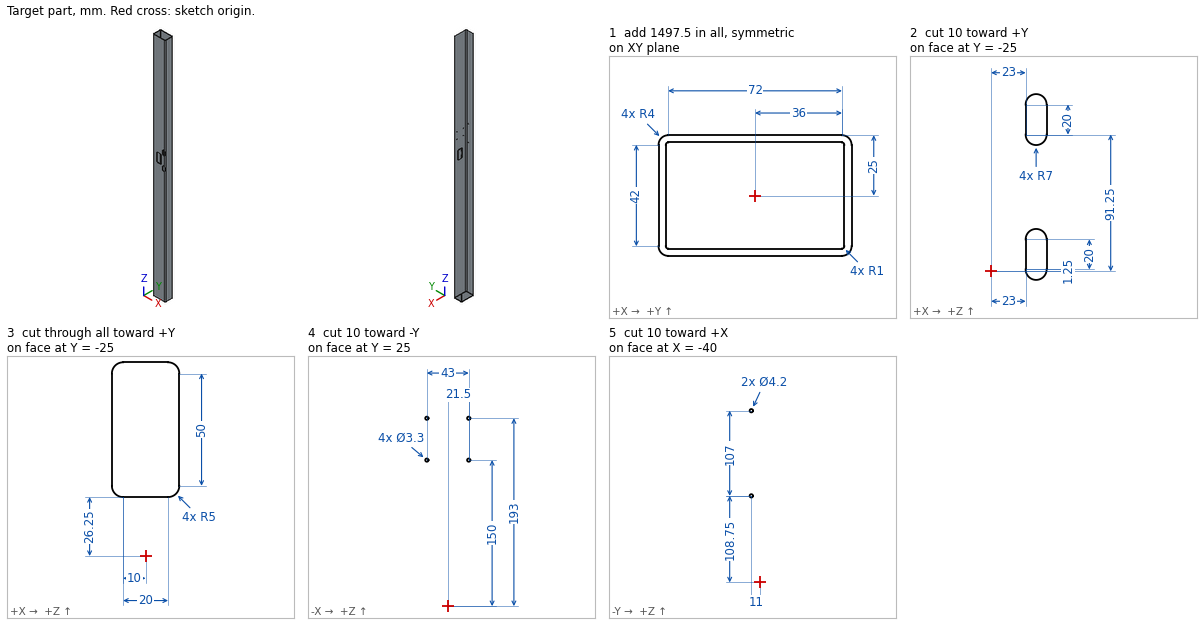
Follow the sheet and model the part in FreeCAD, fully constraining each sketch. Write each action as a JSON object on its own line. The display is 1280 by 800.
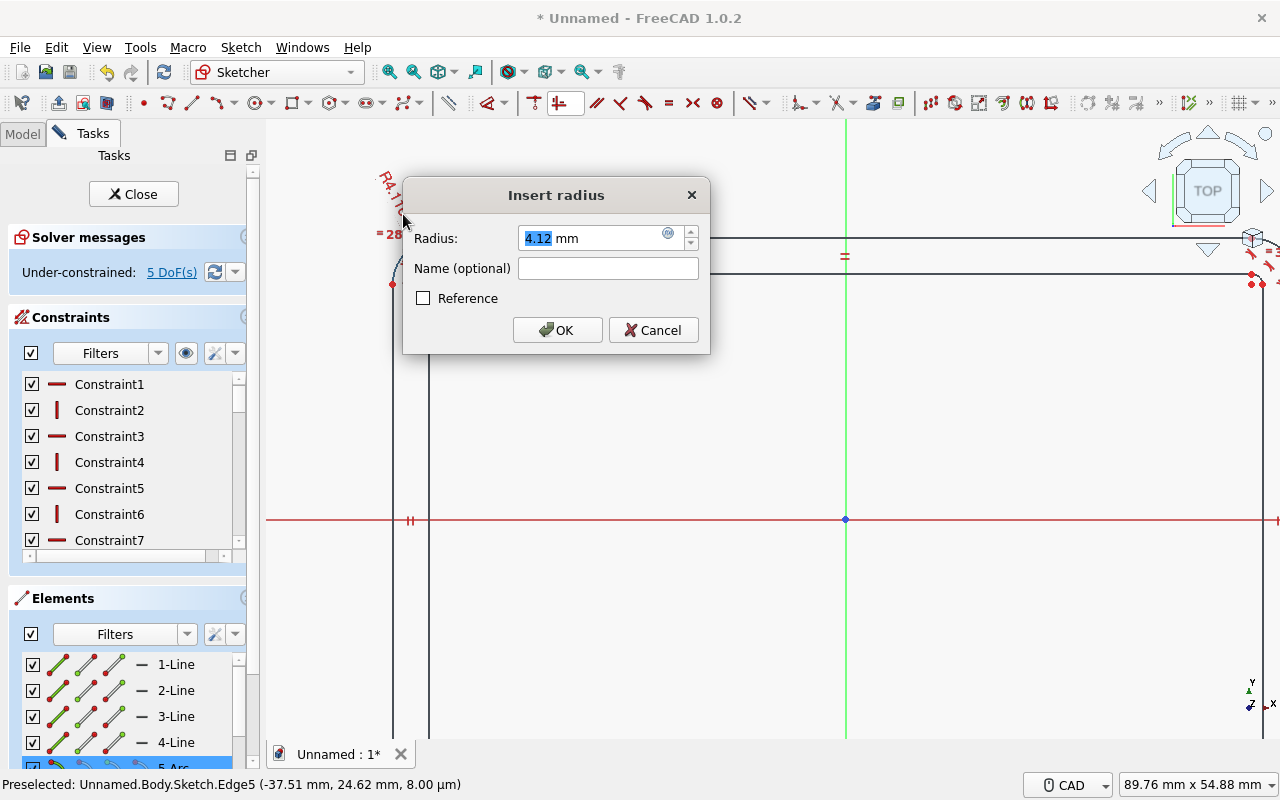
{"action": "type", "text": "4"}
{"action": "key", "text": "Return"}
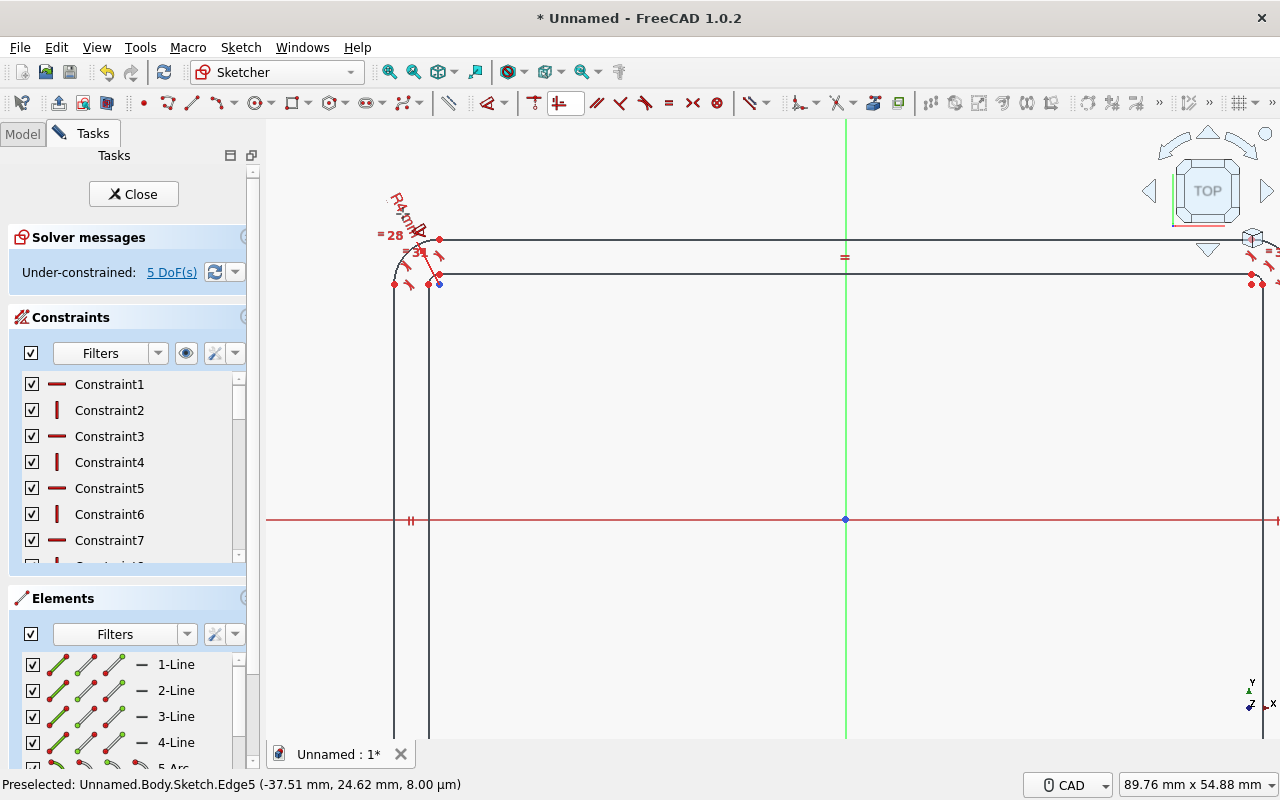
{"action": "scroll", "coordinate": [417, 245], "scroll_direction": "down", "scroll_amount": 2}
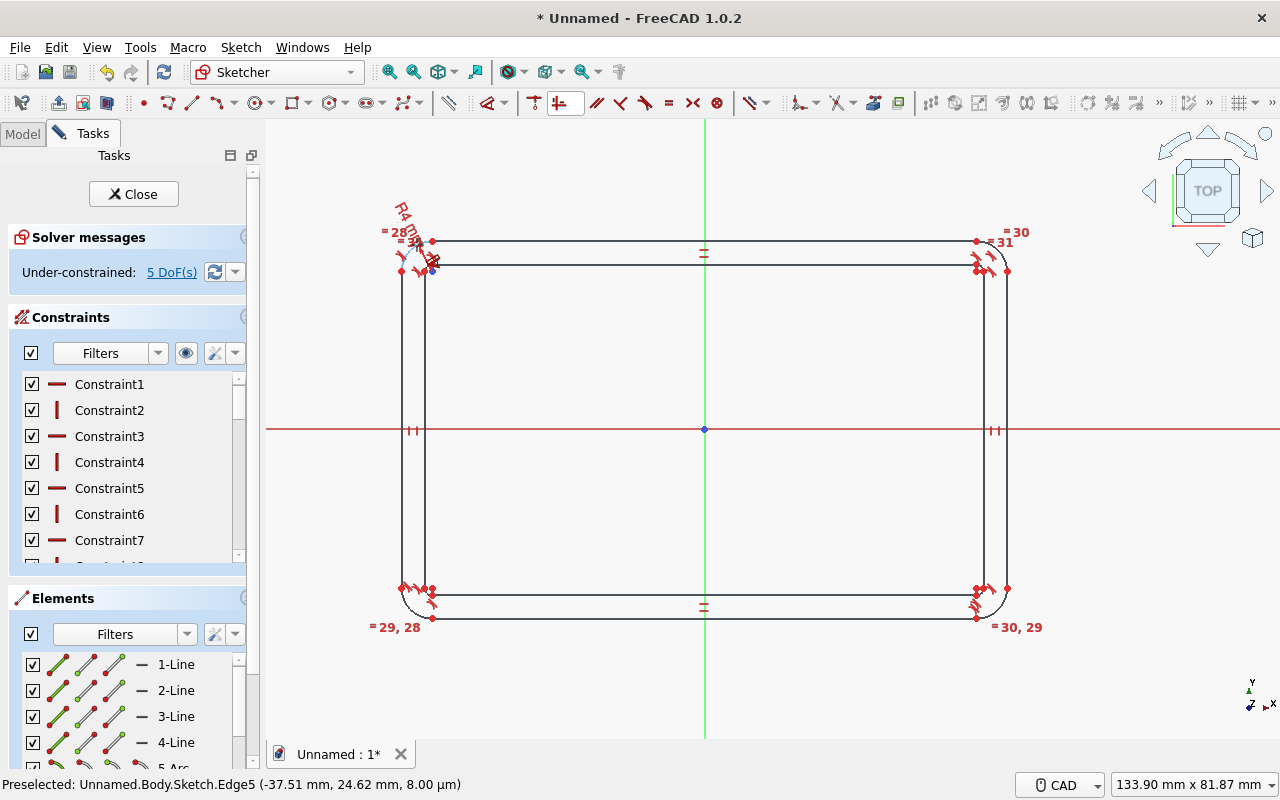
{"action": "scroll", "coordinate": [982, 267], "scroll_direction": "up", "scroll_amount": 9}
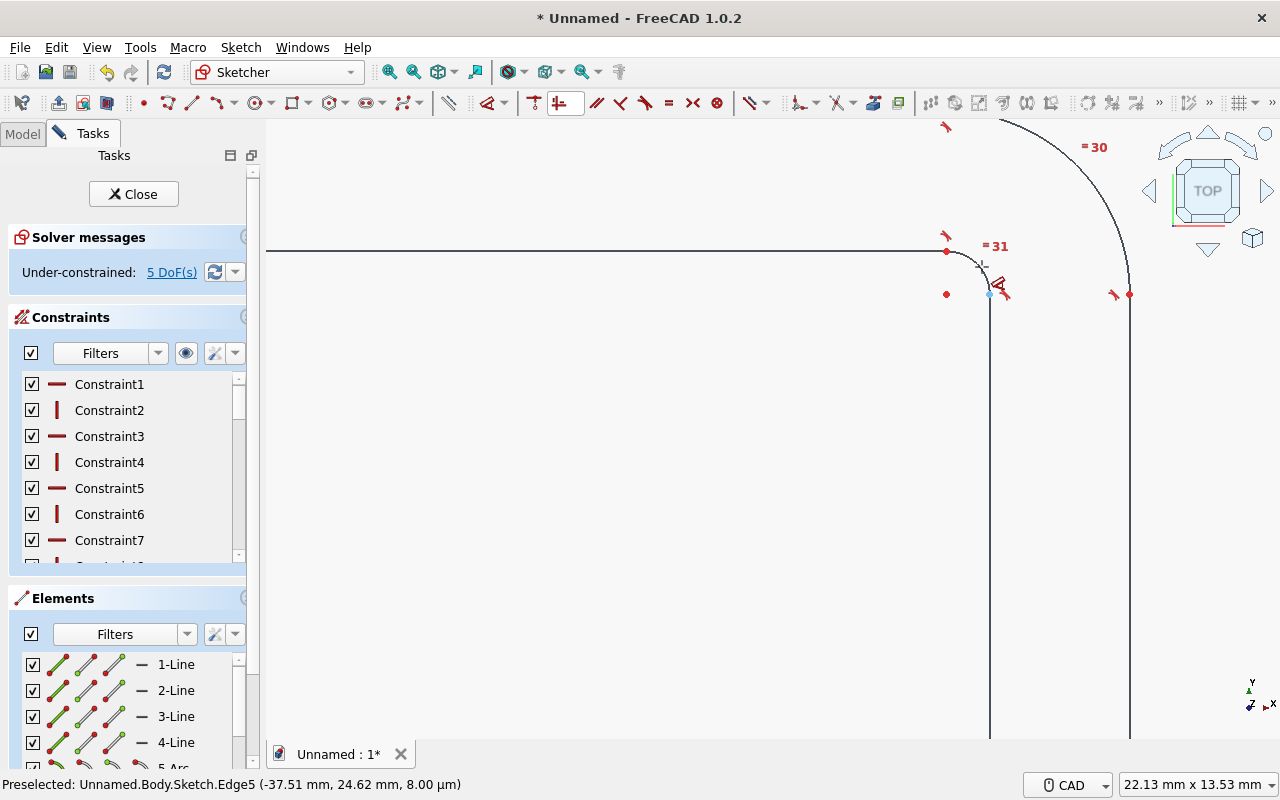
{"action": "left_click", "coordinate": [977, 264]}
{"action": "left_click", "coordinate": [1000, 241]}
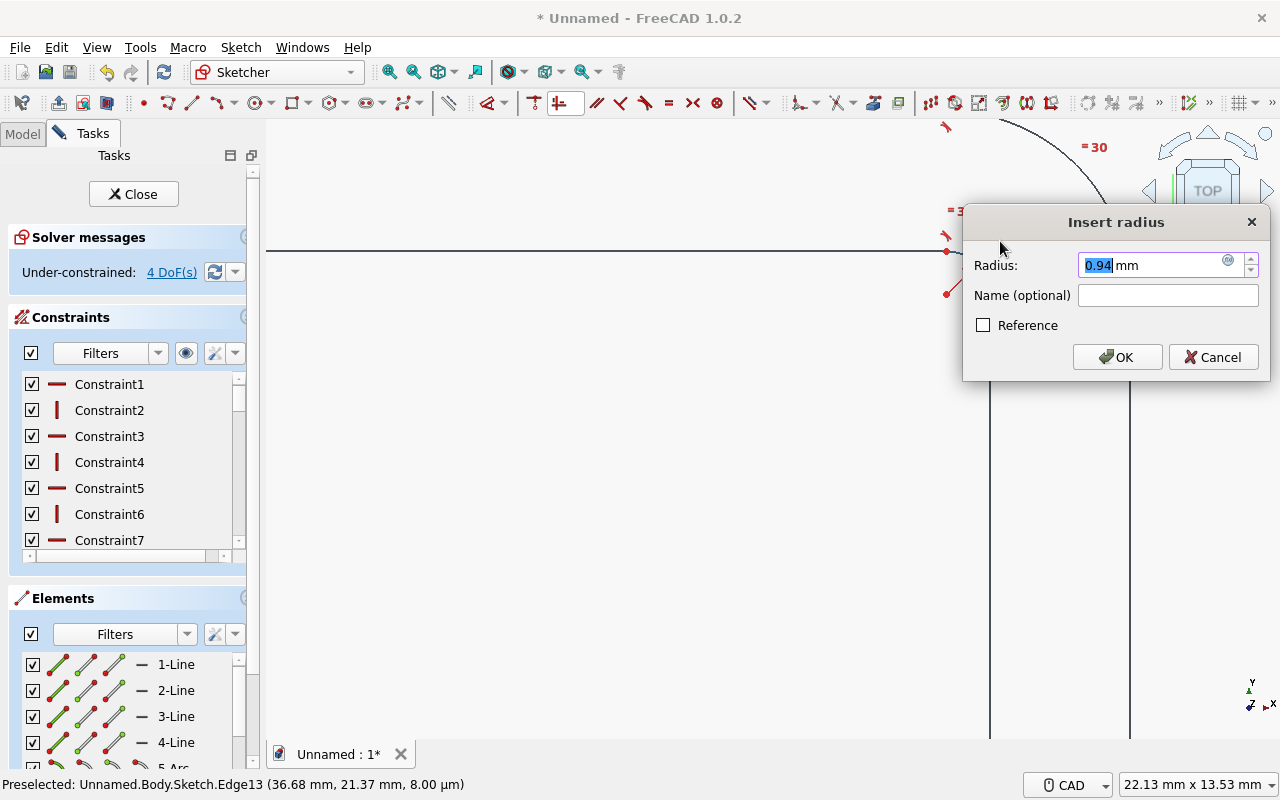
{"action": "type", "text": "1"}
{"action": "key", "text": "Return"}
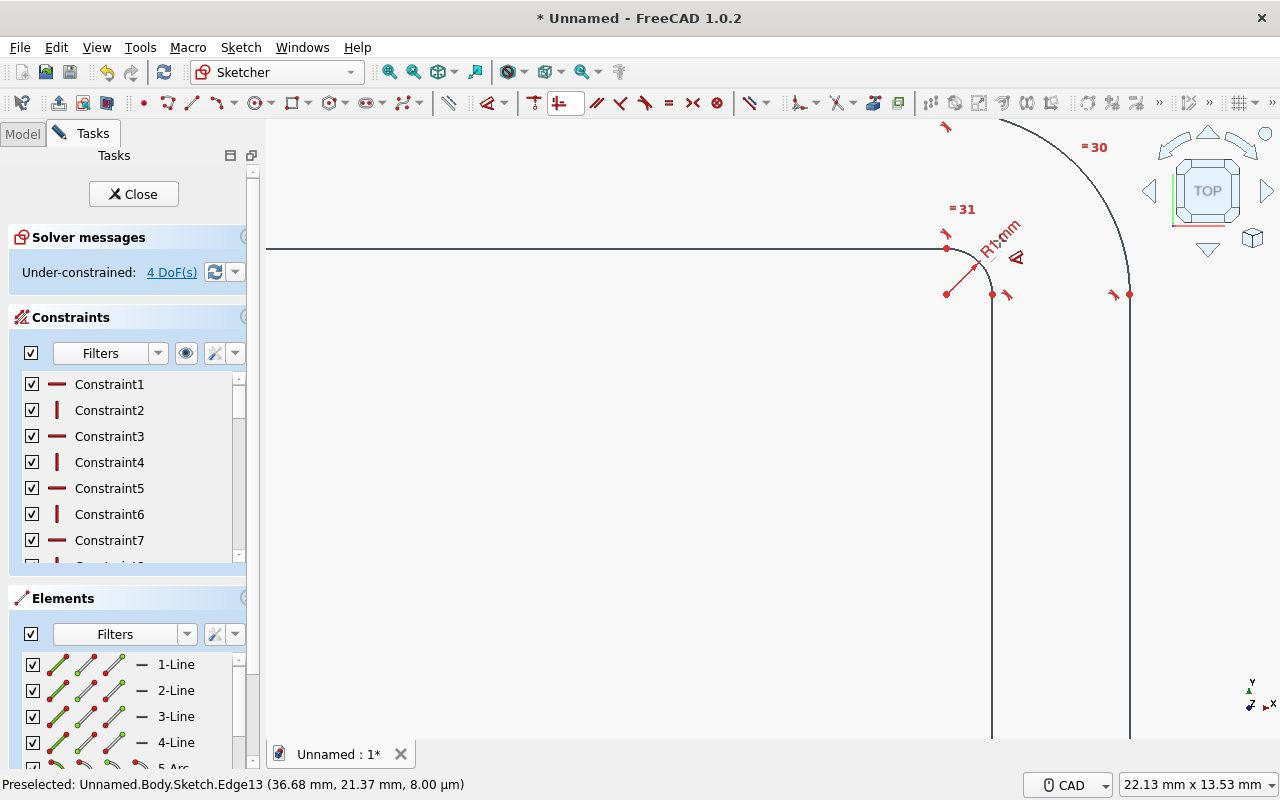
{"action": "scroll", "coordinate": [983, 267], "scroll_direction": "down", "scroll_amount": 9}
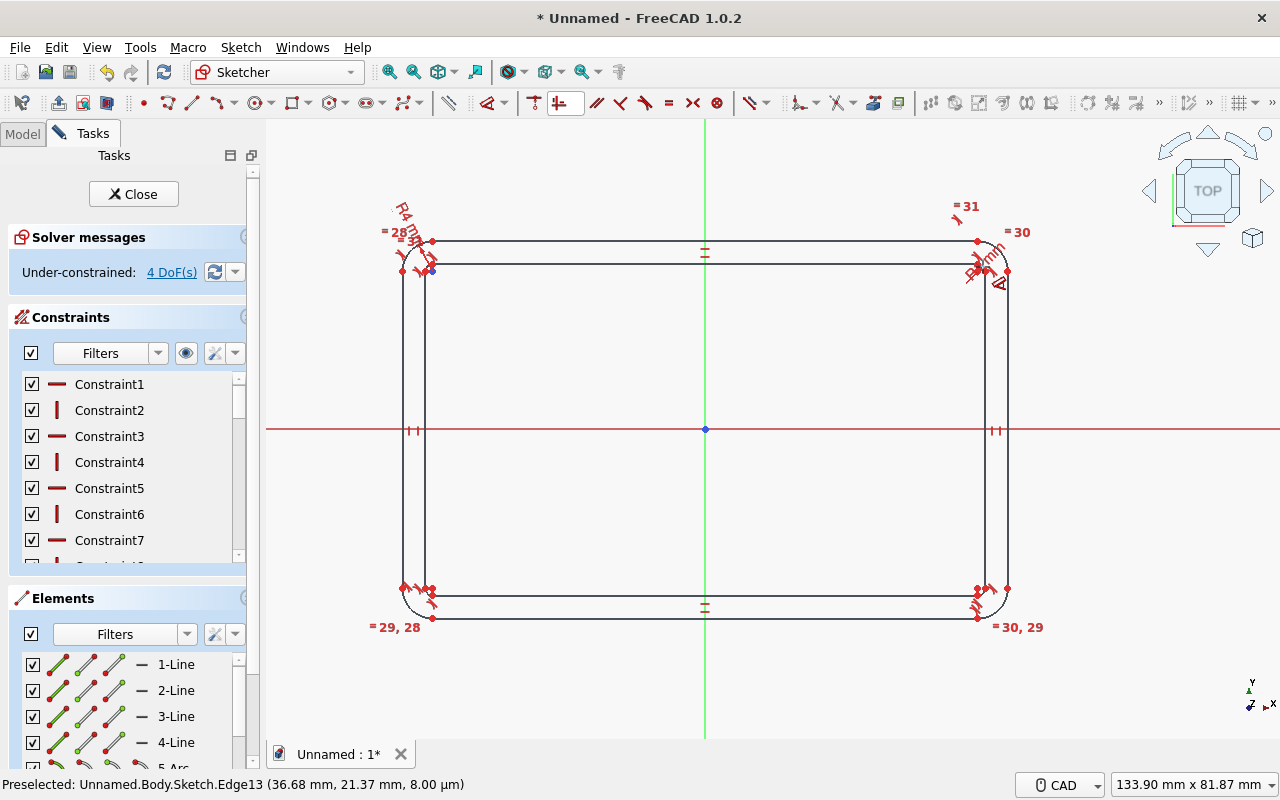
{"action": "left_click", "coordinate": [814, 241]}
{"action": "left_click", "coordinate": [580, 207]}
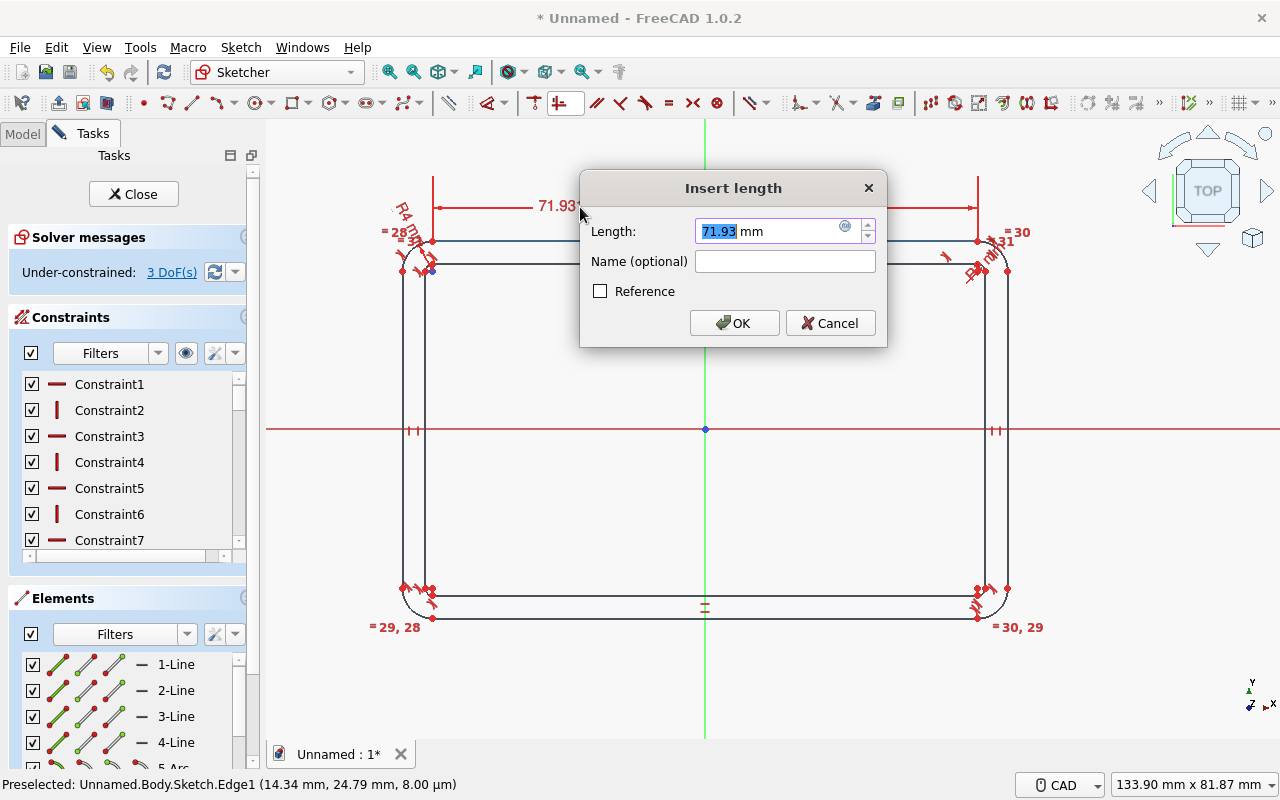
{"action": "type", "text": "72"}
{"action": "key", "text": "Return"}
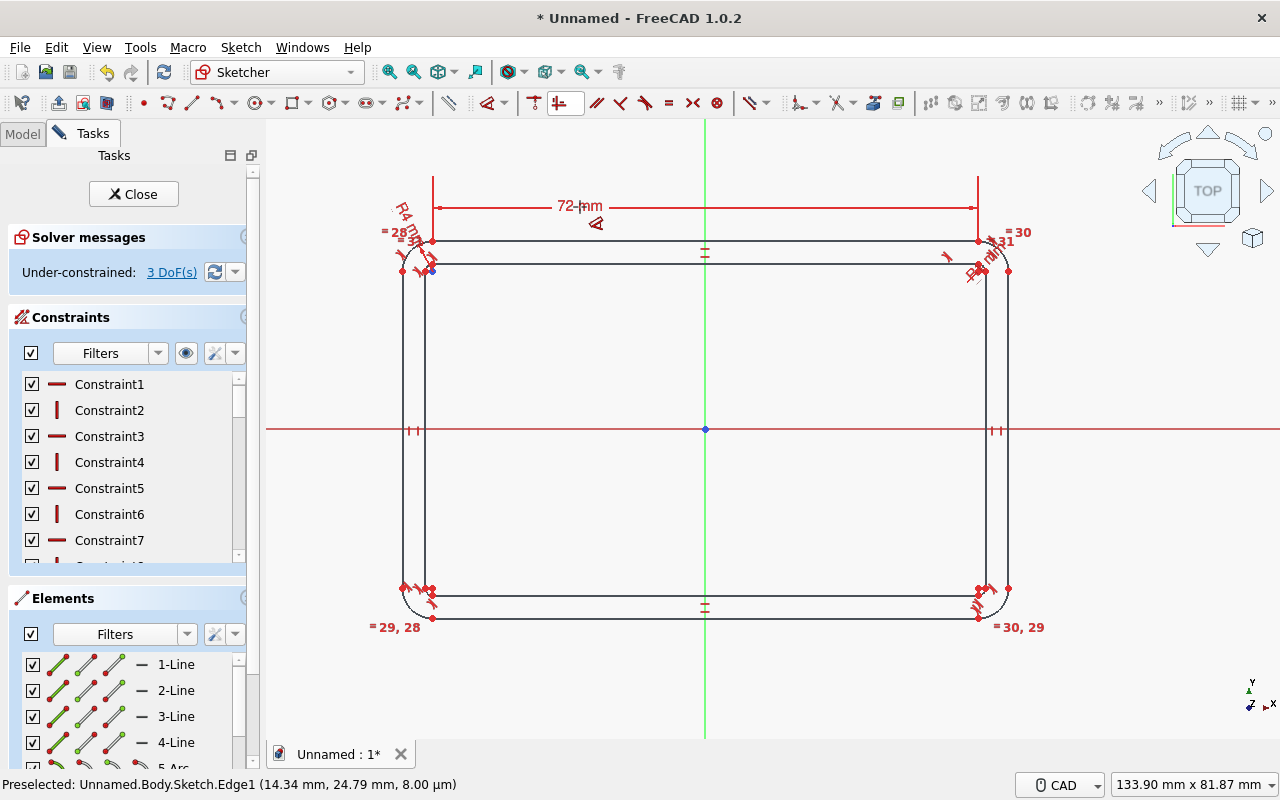
{"action": "left_click", "coordinate": [403, 367]}
{"action": "left_click", "coordinate": [369, 357]}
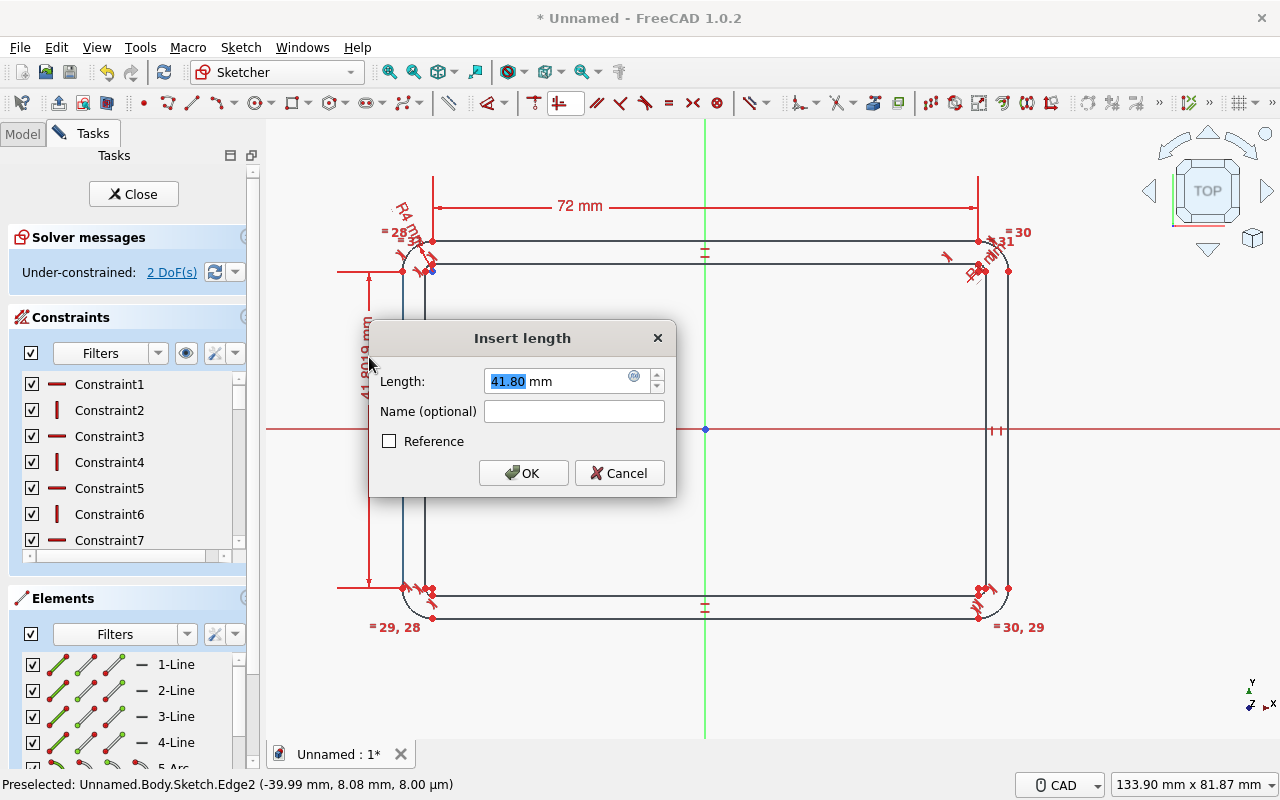
{"action": "type", "text": "42"}
{"action": "key", "text": "Return"}